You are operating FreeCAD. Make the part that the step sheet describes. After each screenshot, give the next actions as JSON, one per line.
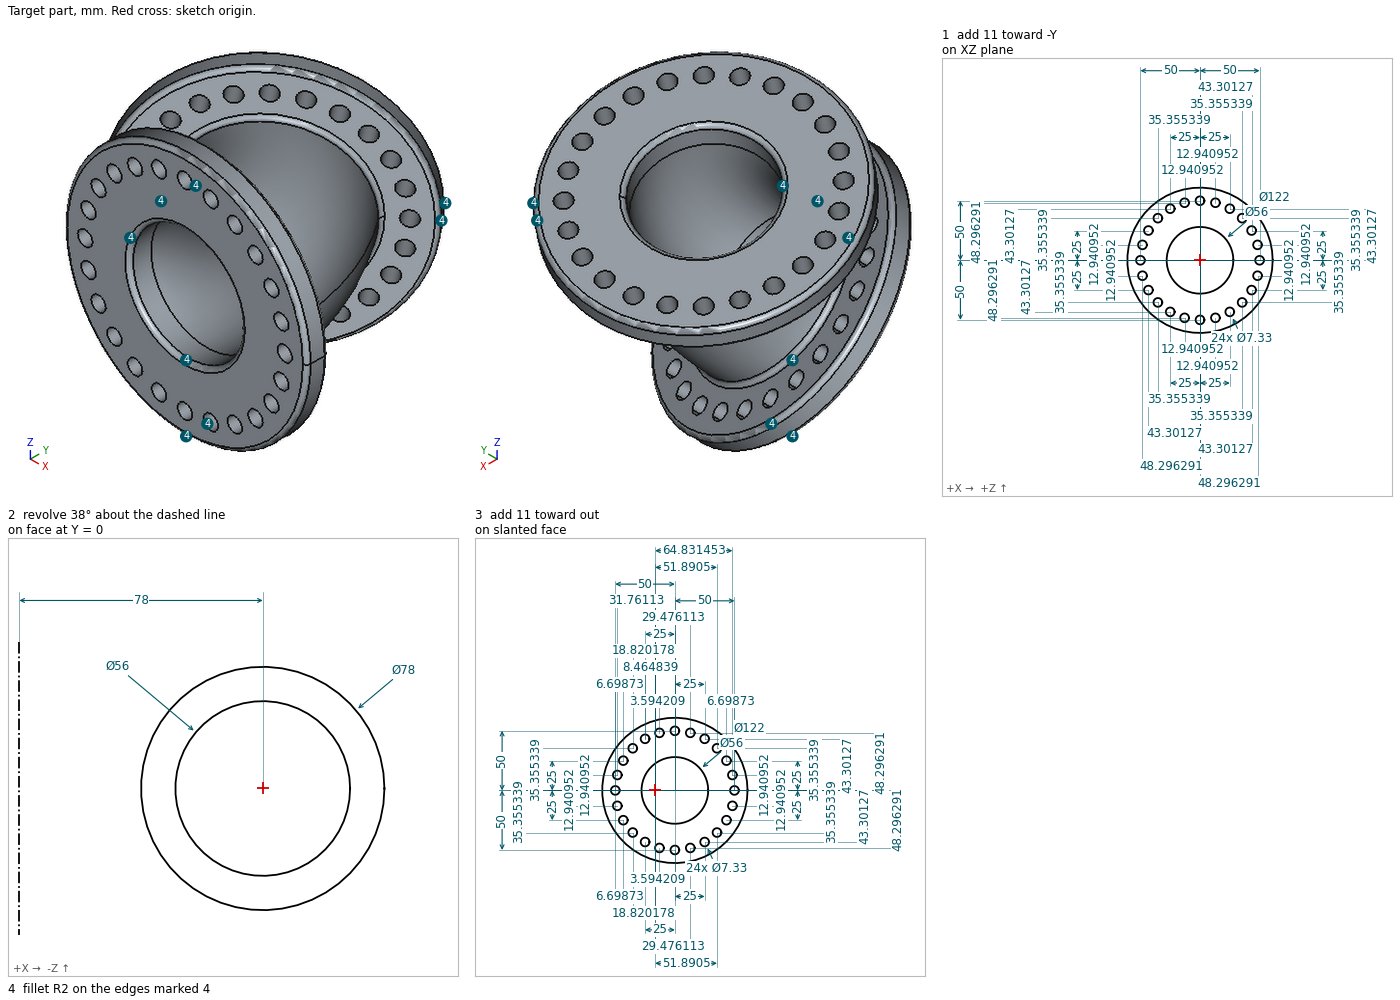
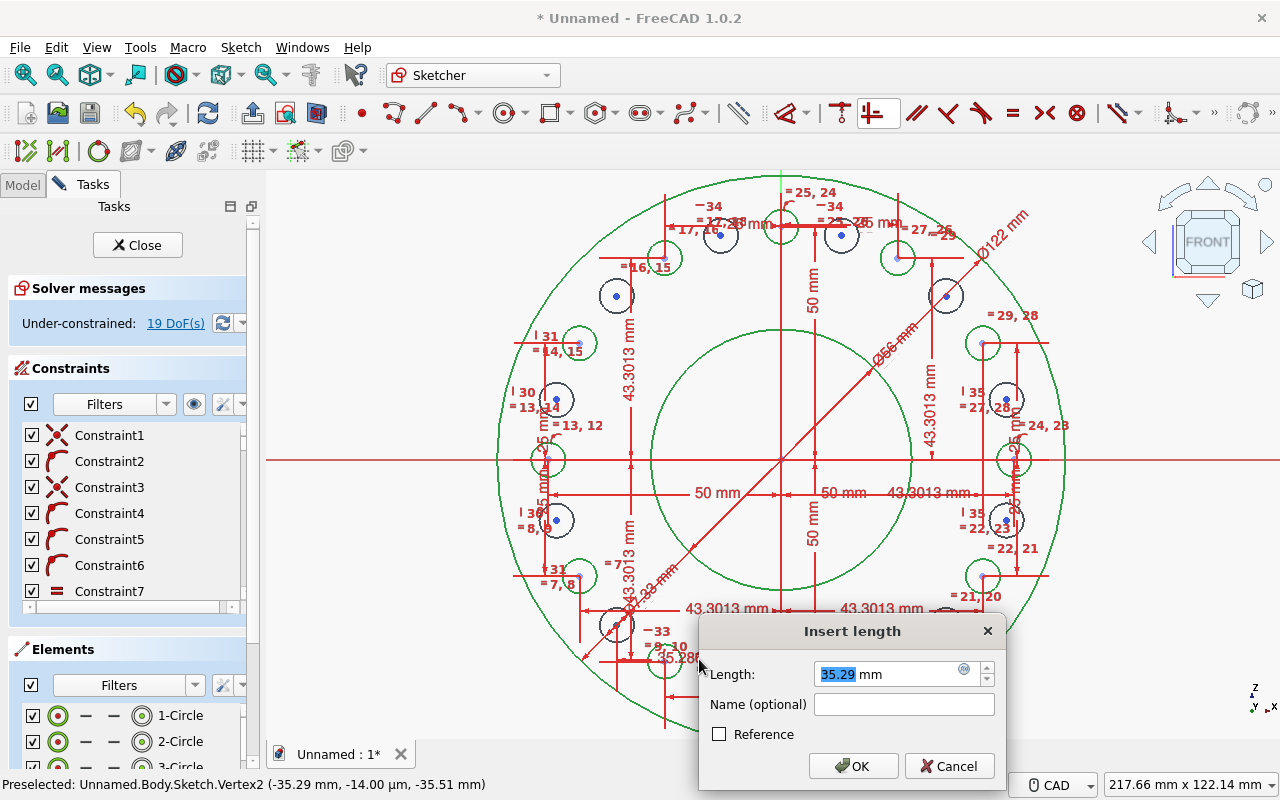
{"action": "type", "text": "35.355339"}
{"action": "key", "text": "Return"}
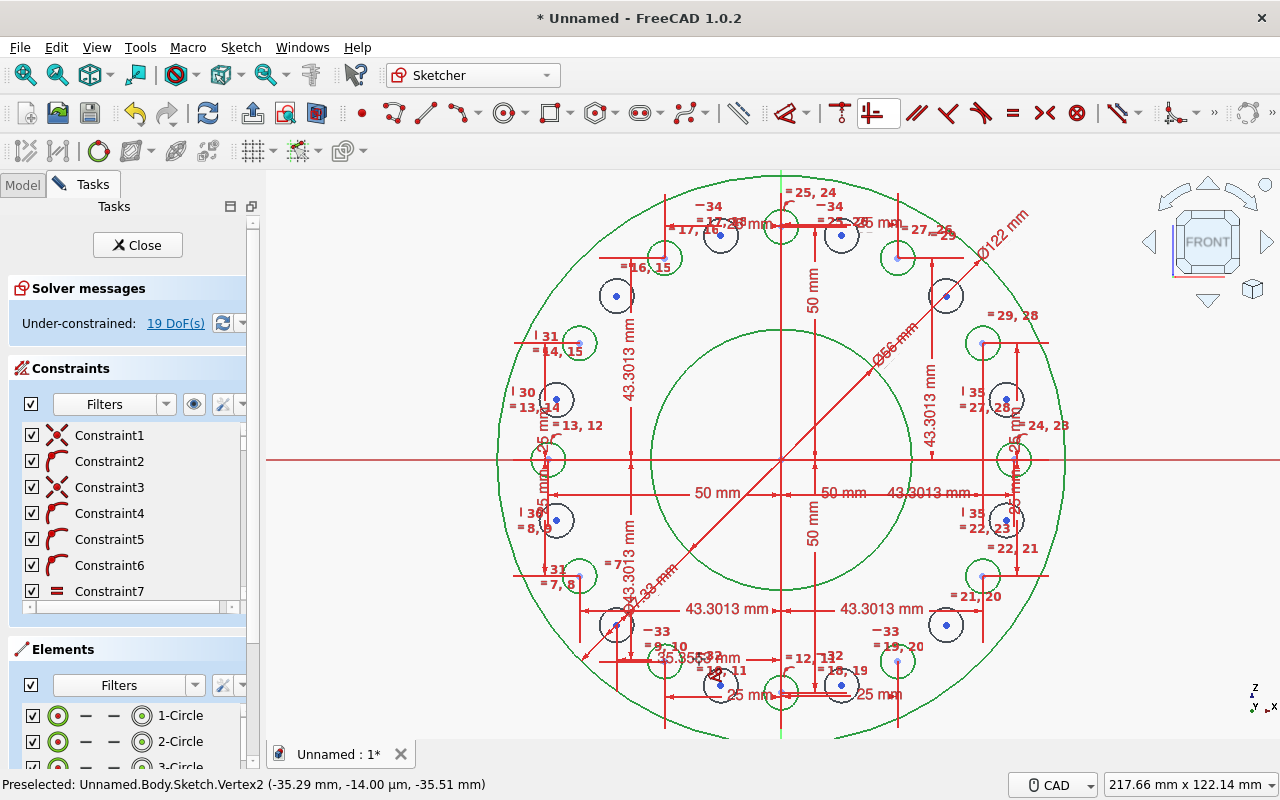
{"action": "left_click", "coordinate": [617, 625]}
{"action": "left_click", "coordinate": [559, 600]}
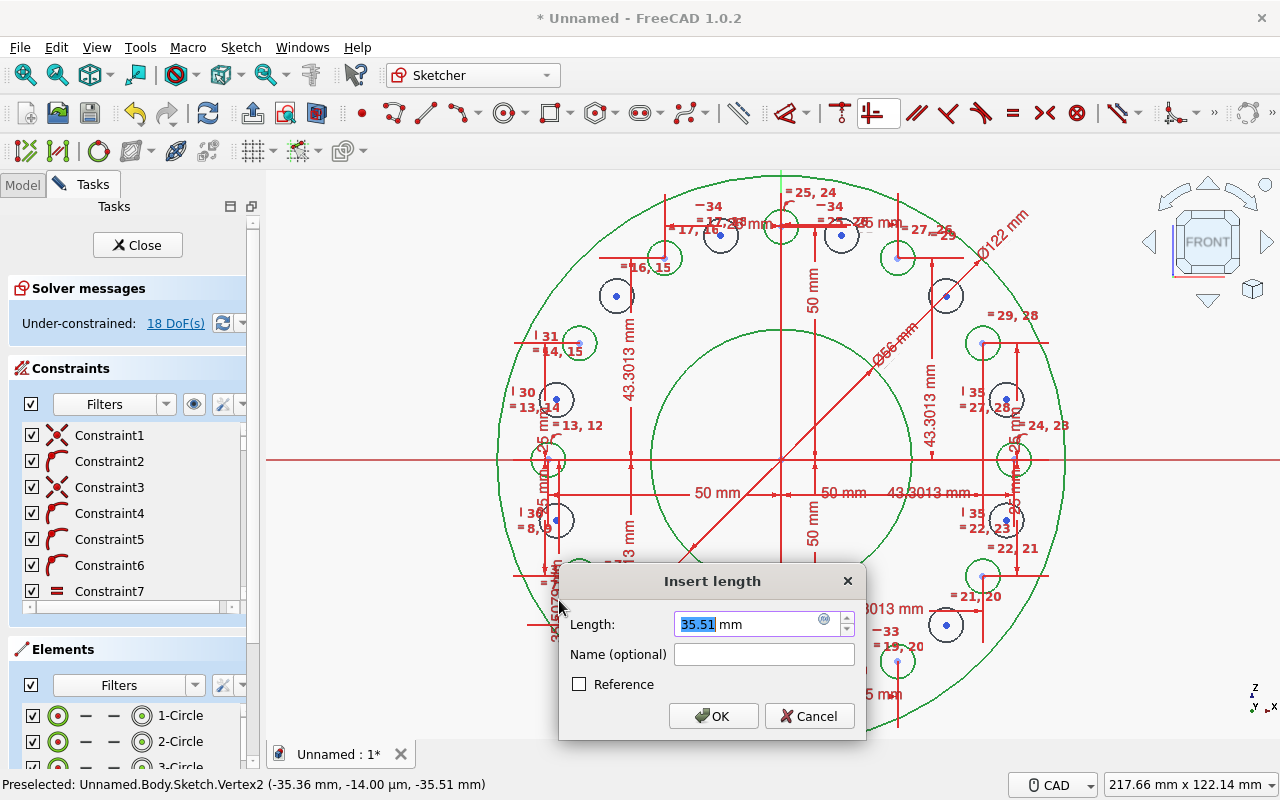
{"action": "type", "text": "35.355339"}
{"action": "key", "text": "Return"}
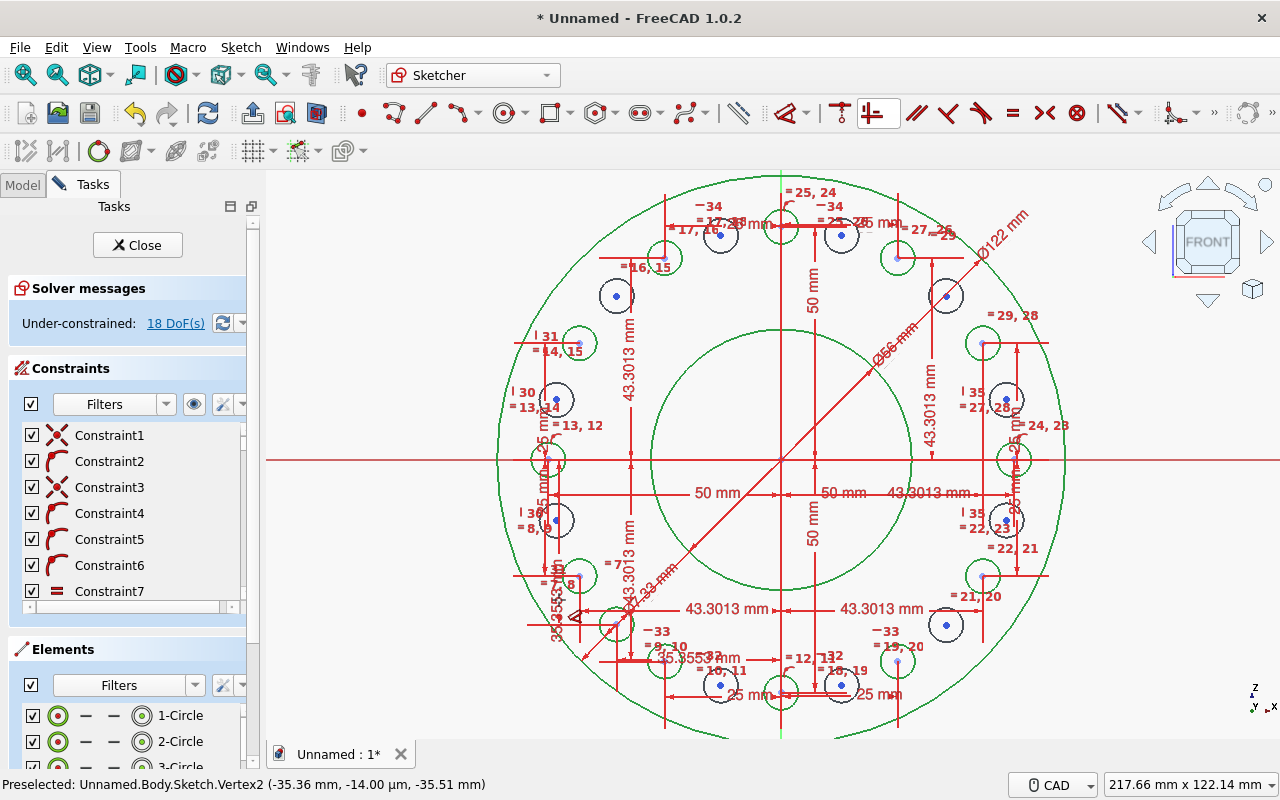
{"action": "left_click", "coordinate": [557, 521]}
{"action": "left_click", "coordinate": [721, 555]}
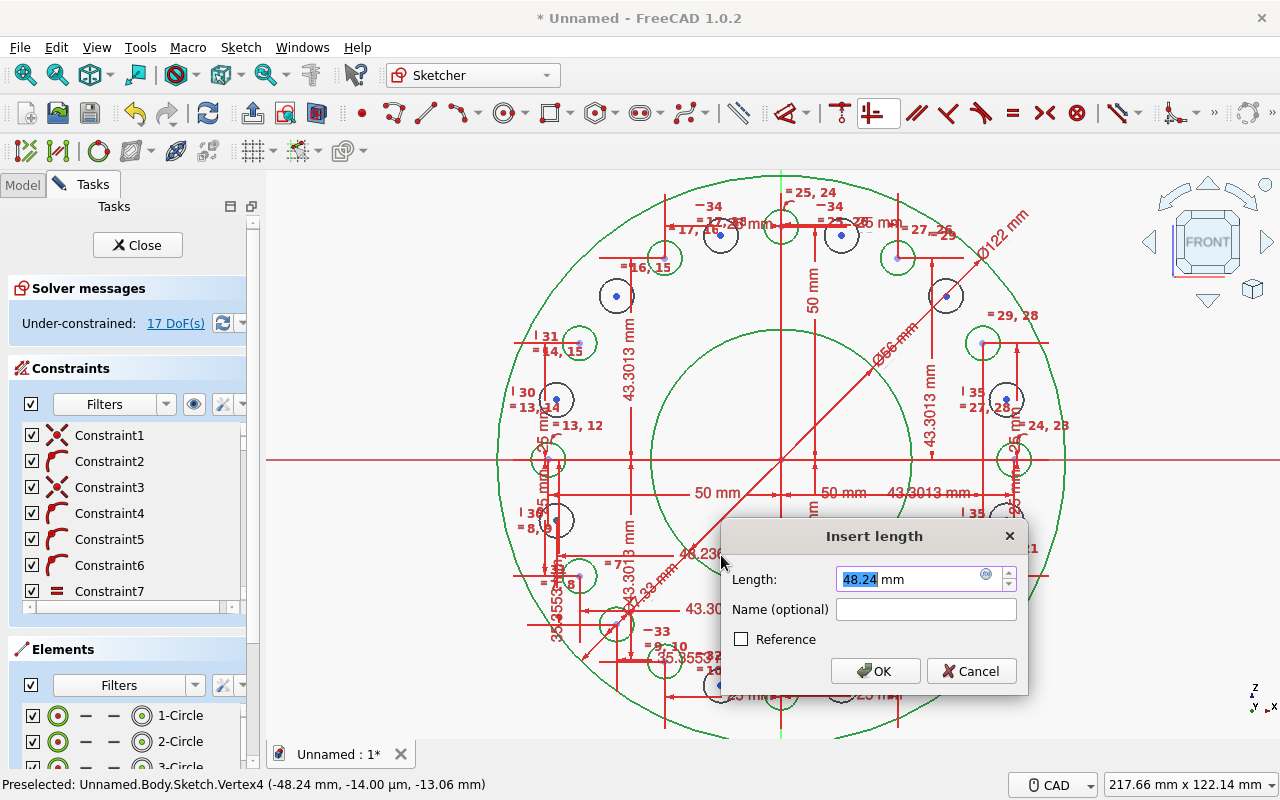
{"action": "type", "text": "48.296291"}
{"action": "key", "text": "Return"}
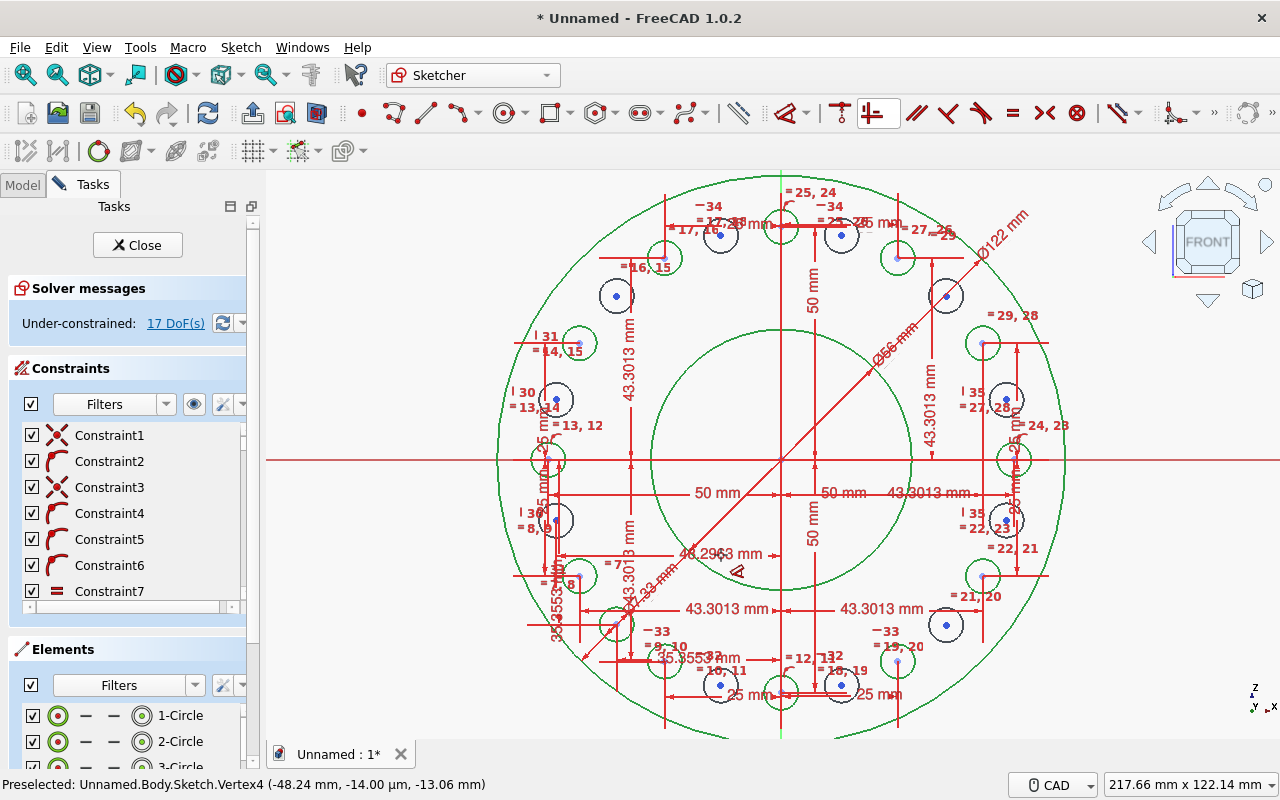
{"action": "left_click", "coordinate": [556, 521]}
{"action": "left_click", "coordinate": [522, 512]}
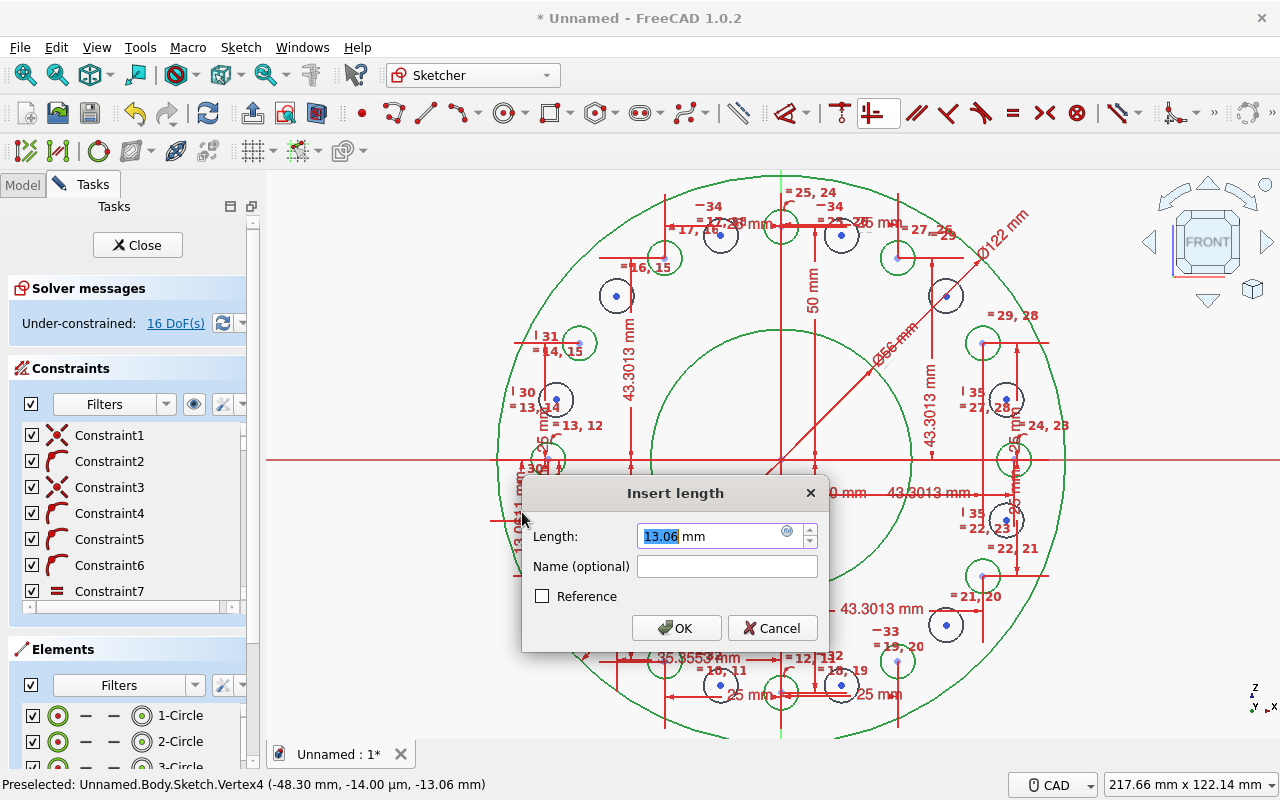
{"action": "type", "text": "12.940952"}
{"action": "key", "text": "Return"}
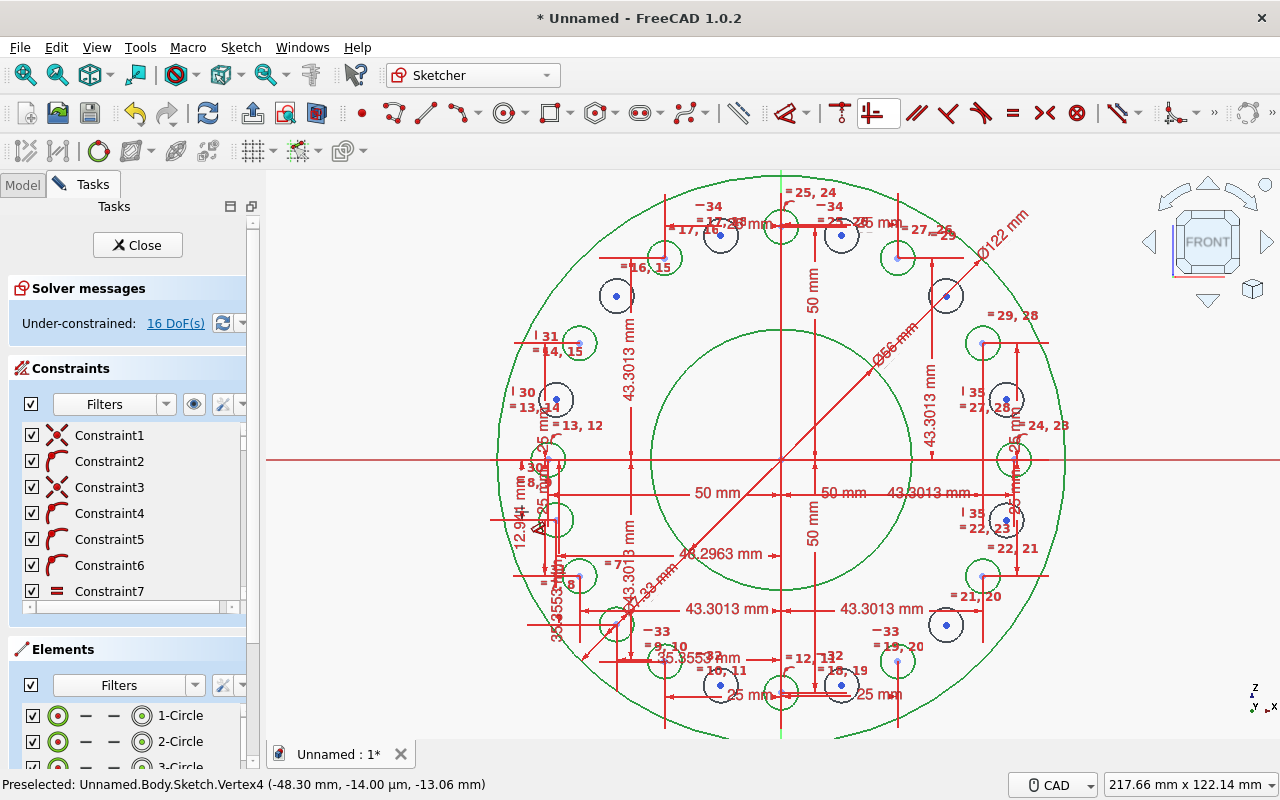
{"action": "left_click", "coordinate": [721, 686]}
{"action": "left_click", "coordinate": [751, 426]}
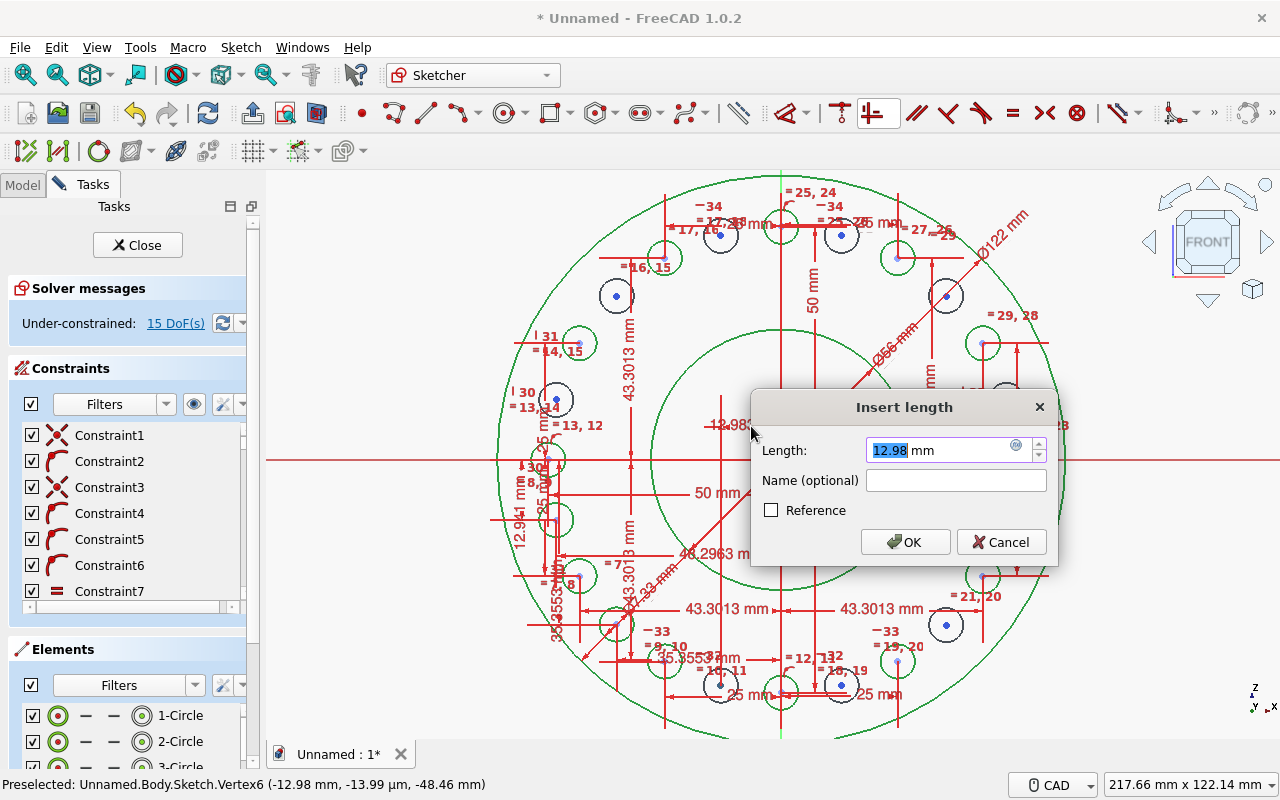
{"action": "type", "text": "12.940952"}
{"action": "key", "text": "Return"}